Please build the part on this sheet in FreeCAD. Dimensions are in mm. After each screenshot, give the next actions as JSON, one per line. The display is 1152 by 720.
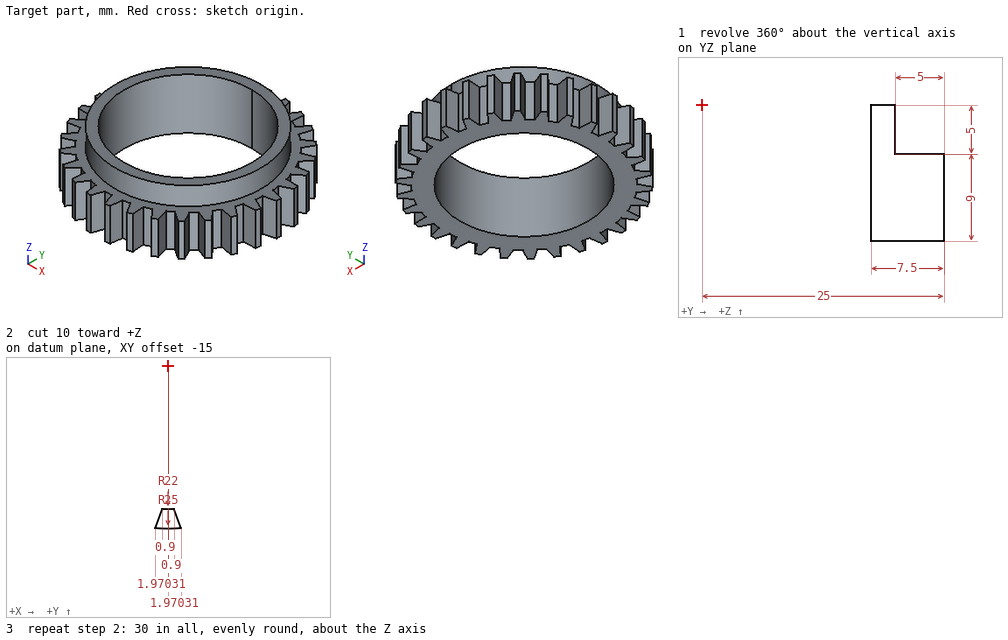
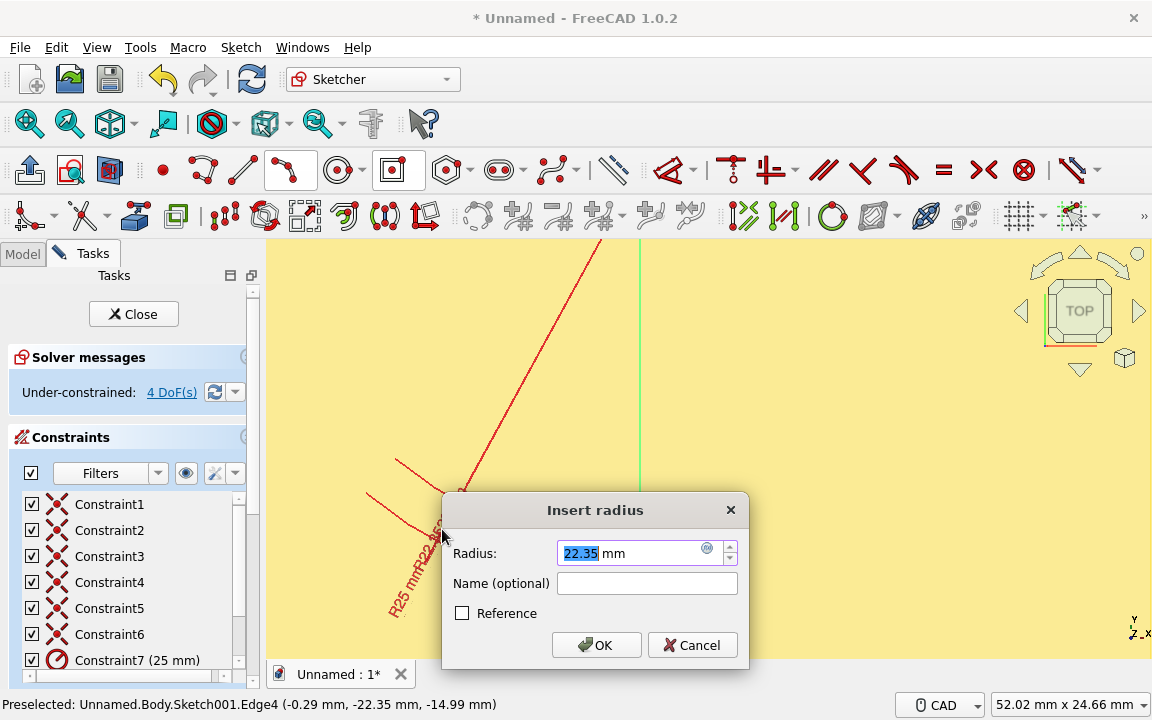
{"action": "type", "text": "22"}
{"action": "key", "text": "Return"}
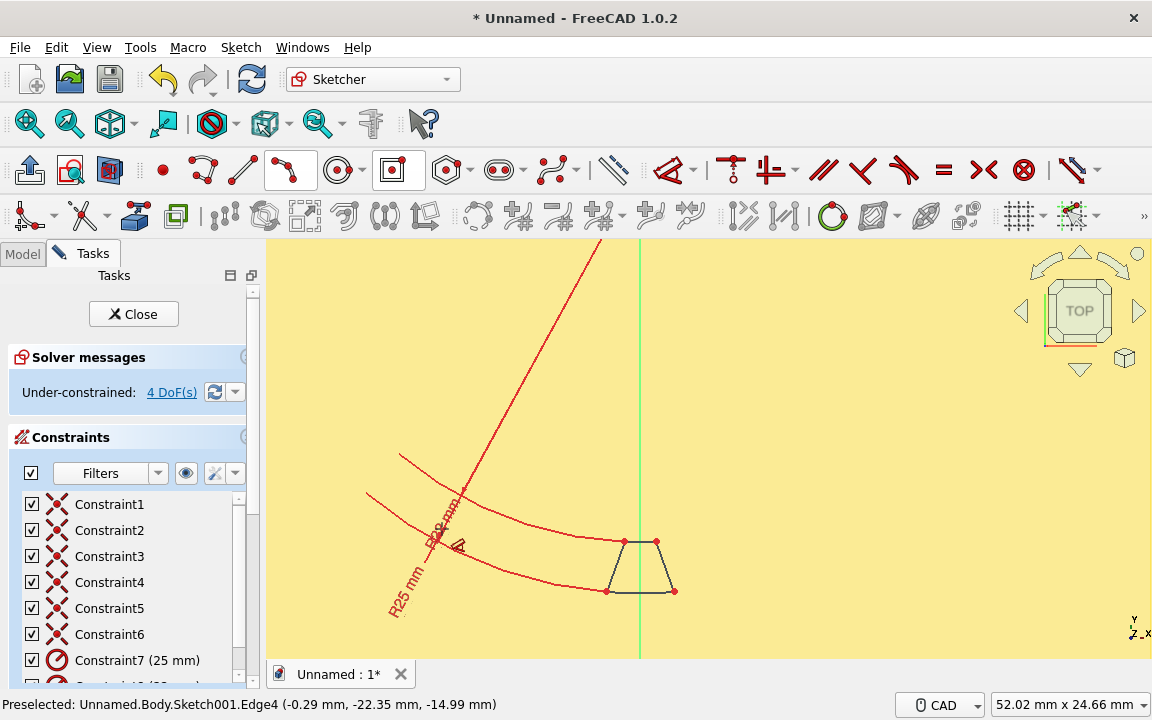
{"action": "scroll", "coordinate": [625, 542], "scroll_direction": "up", "scroll_amount": 5}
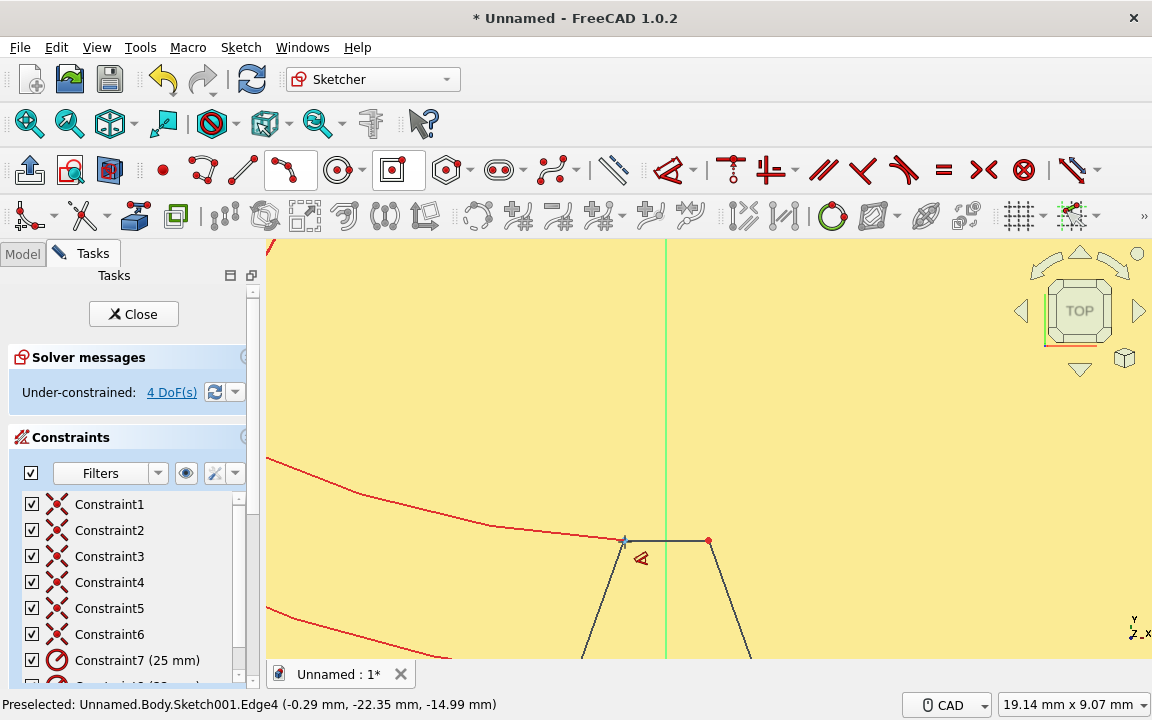
{"action": "left_click", "coordinate": [624, 540]}
{"action": "left_click", "coordinate": [645, 574]}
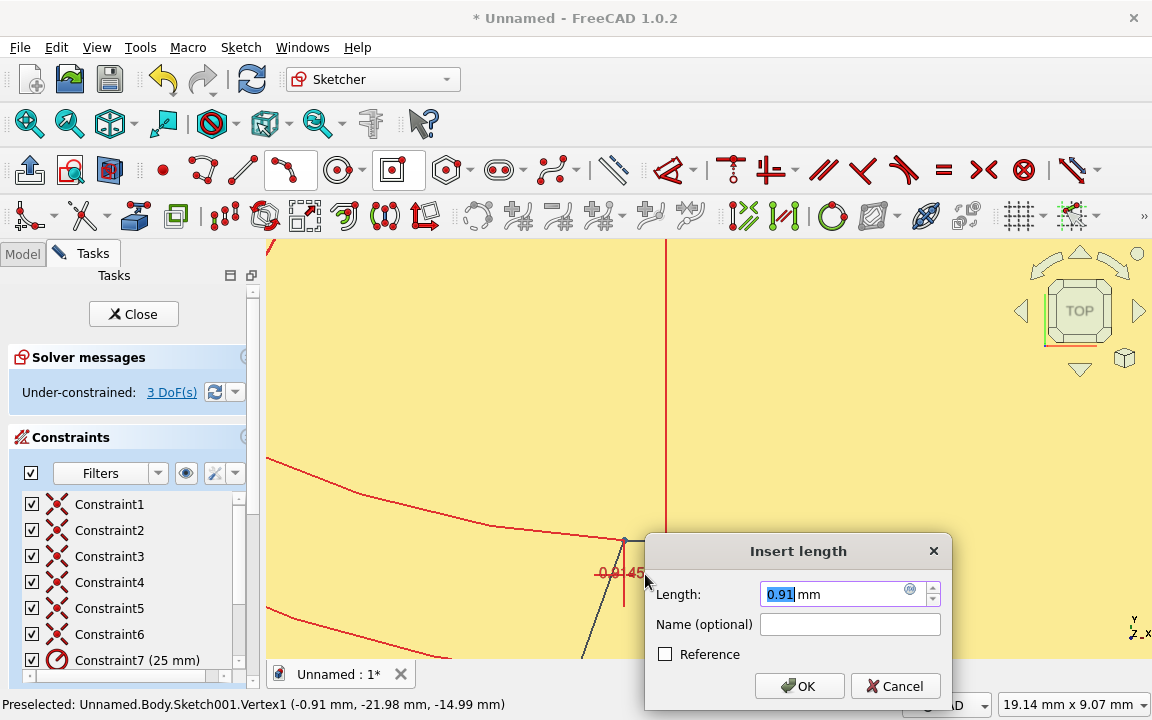
{"action": "type", "text": "0.9"}
{"action": "key", "text": "Return"}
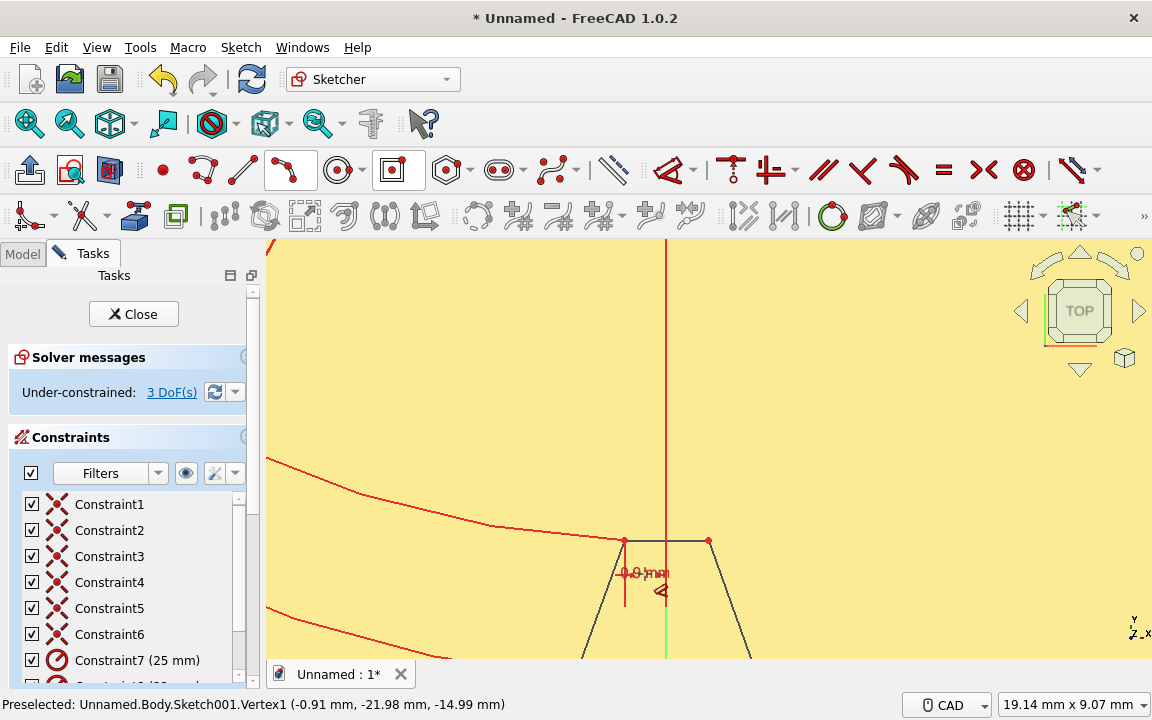
{"action": "left_click", "coordinate": [709, 540]}
{"action": "left_click", "coordinate": [688, 598]}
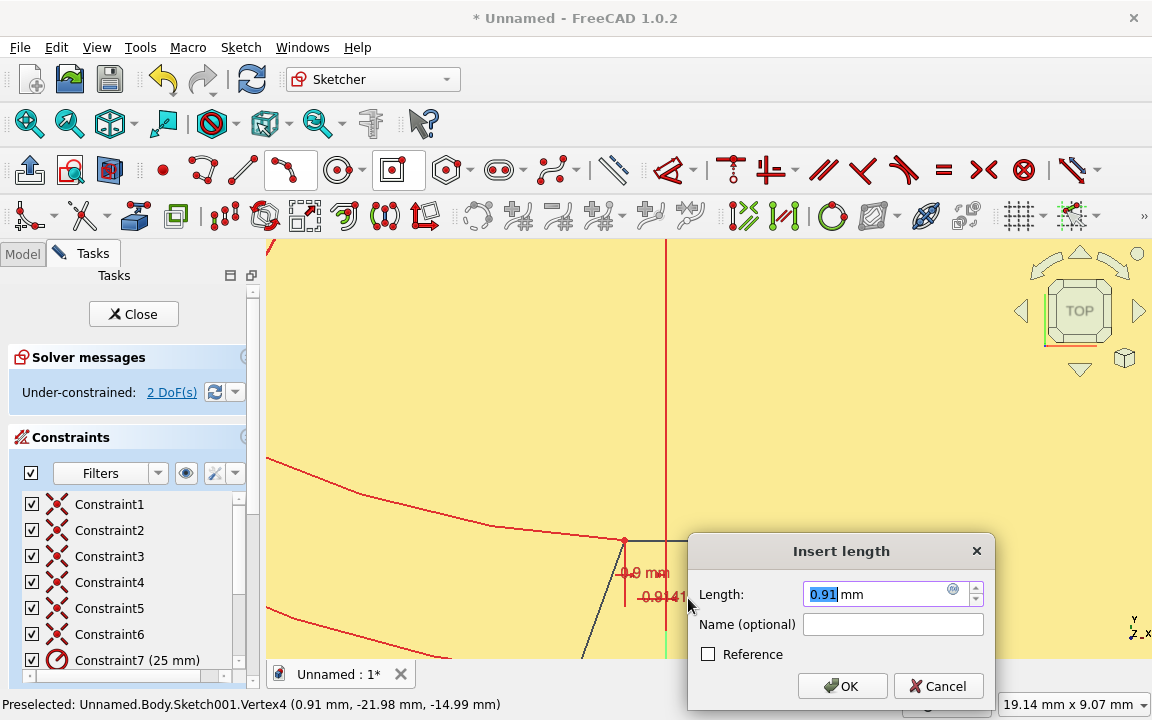
{"action": "type", "text": "0.9"}
{"action": "key", "text": "Return"}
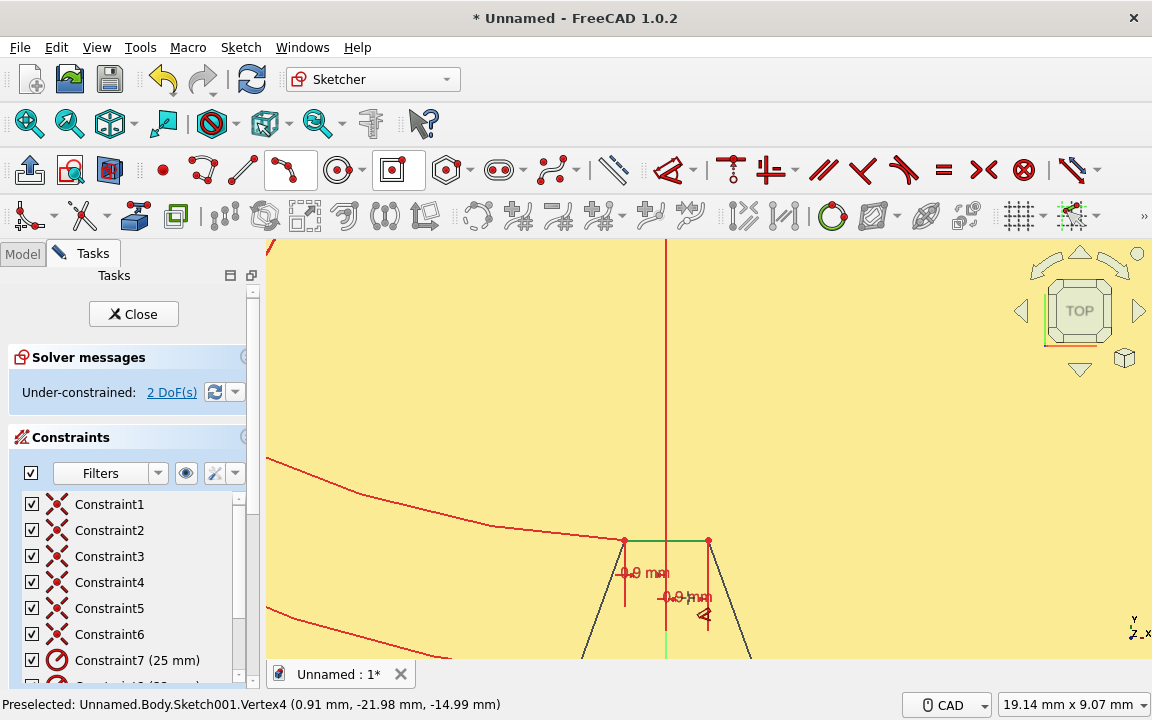
{"action": "scroll", "coordinate": [640, 449], "scroll_direction": "down", "scroll_amount": 5}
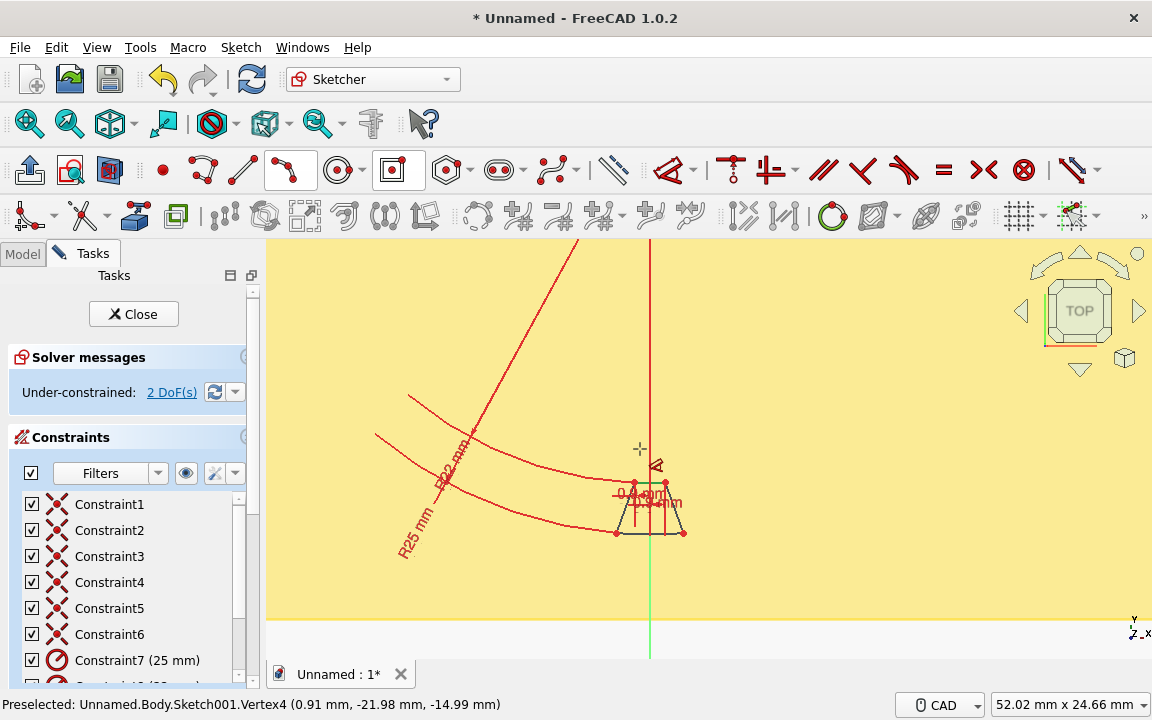
{"action": "scroll", "coordinate": [652, 524], "scroll_direction": "up", "scroll_amount": 8}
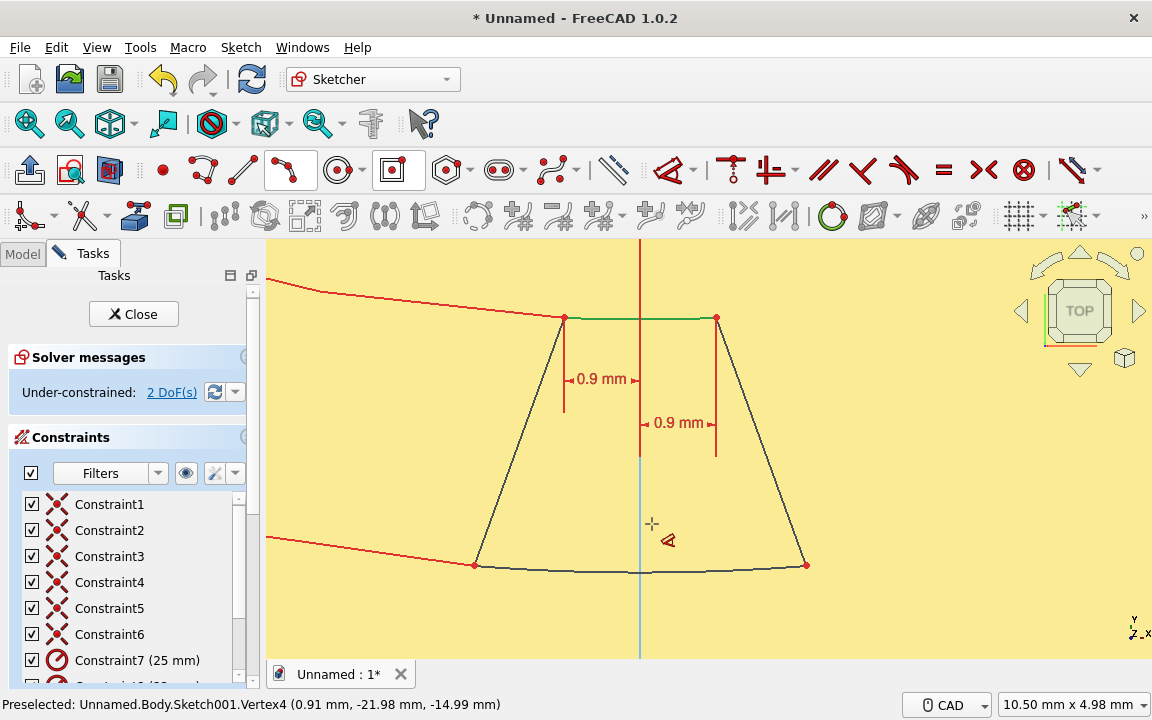
{"action": "left_click", "coordinate": [474, 566]}
{"action": "left_click", "coordinate": [557, 600]}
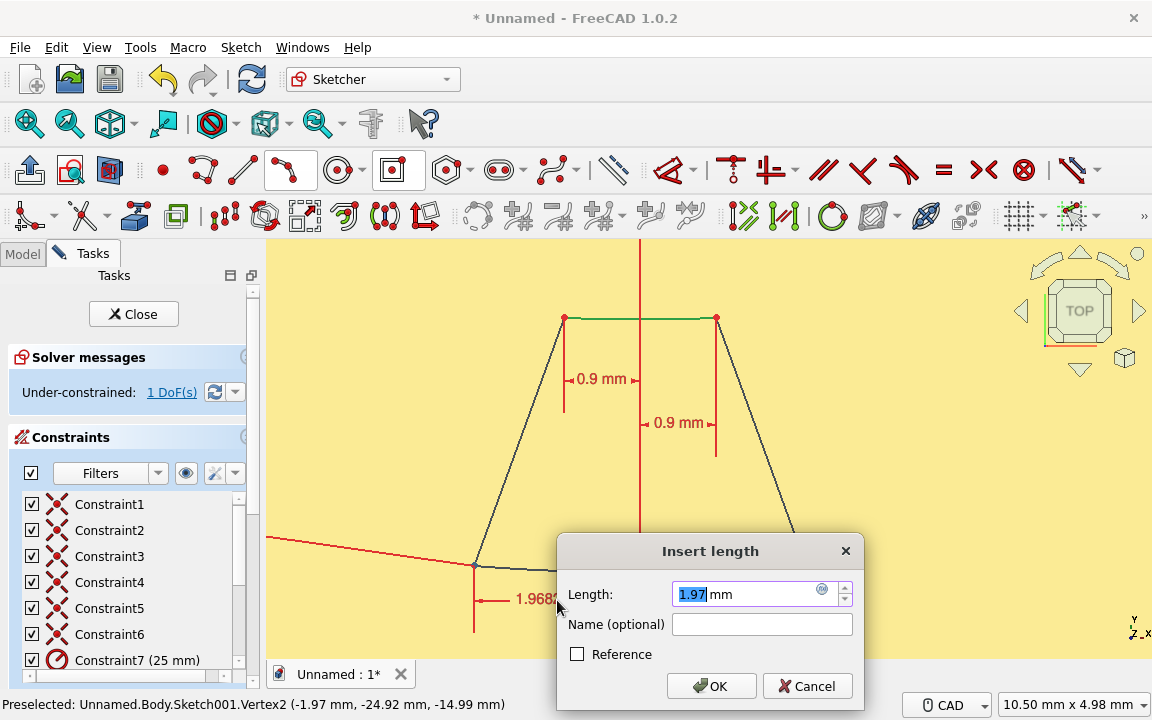
{"action": "type", "text": "1.97031"}
{"action": "key", "text": "Return"}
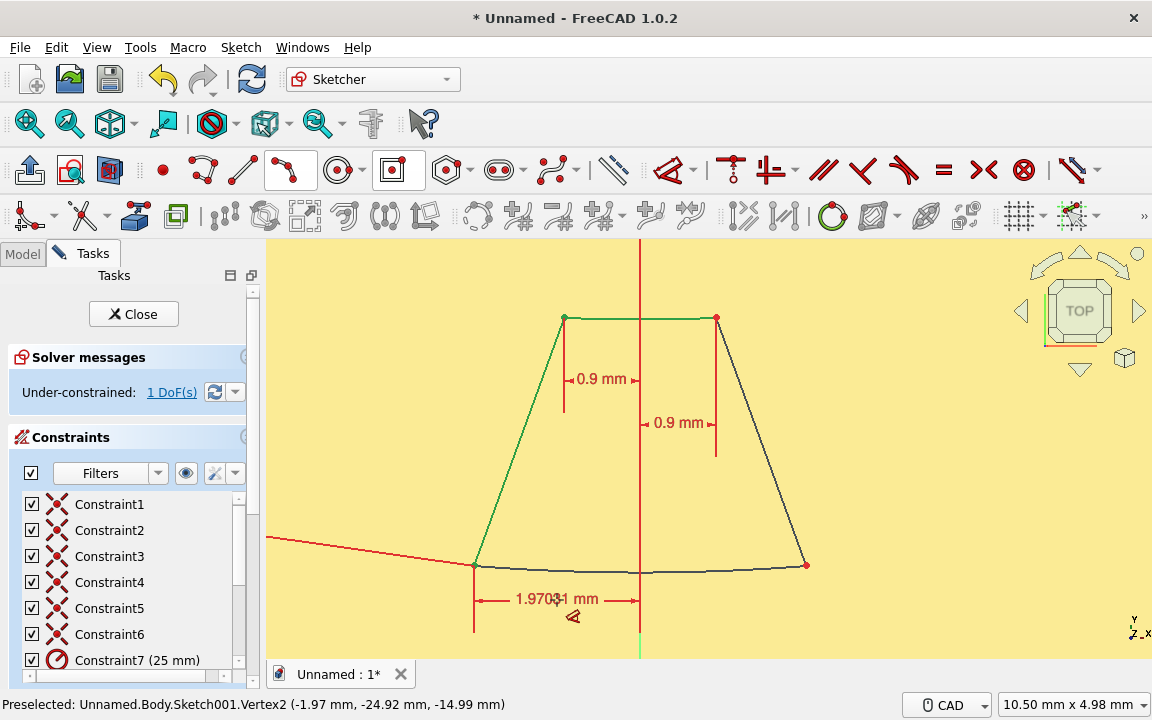
{"action": "left_click", "coordinate": [806, 566]}
{"action": "left_click", "coordinate": [723, 600]}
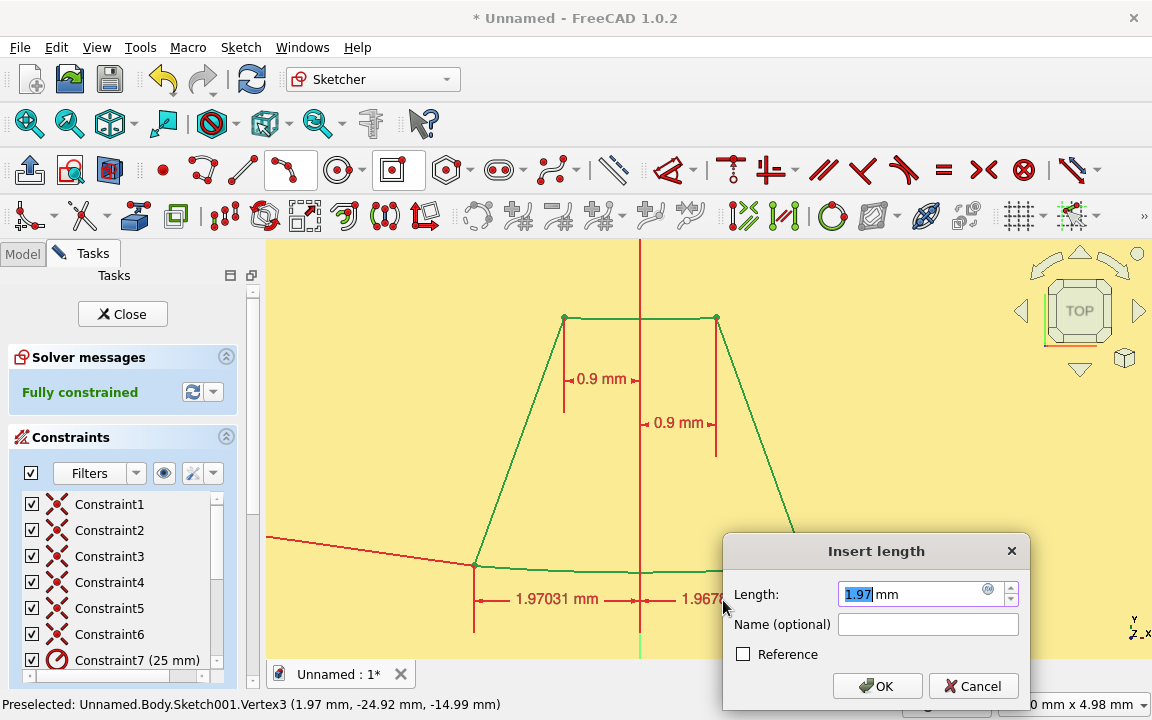
{"action": "type", "text": "1.97031"}
{"action": "key", "text": "Return"}
{"action": "key", "text": "Escape"}